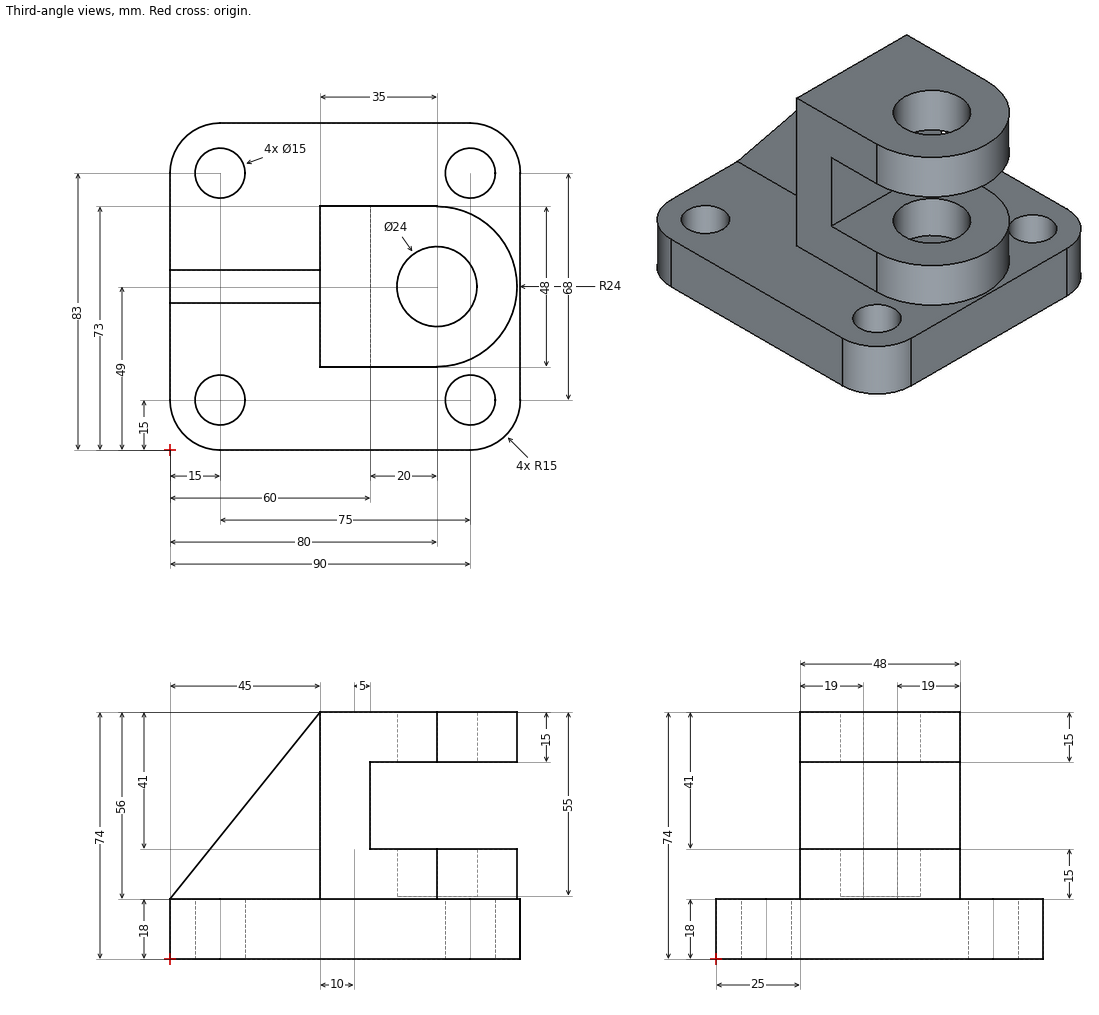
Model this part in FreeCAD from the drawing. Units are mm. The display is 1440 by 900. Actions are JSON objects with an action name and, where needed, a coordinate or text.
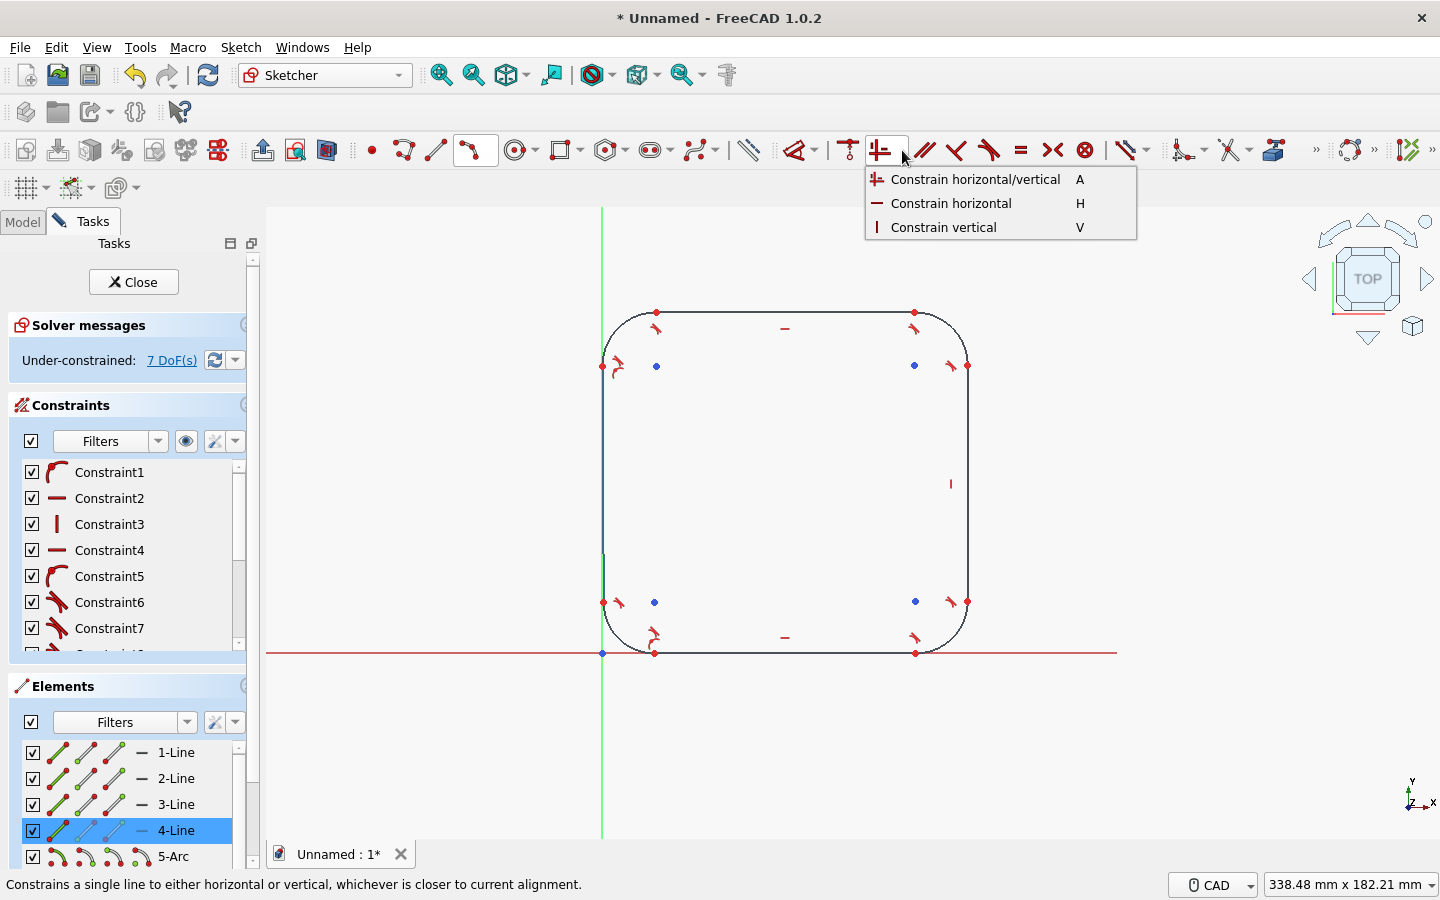
{"action": "left_click", "coordinate": [1001, 227]}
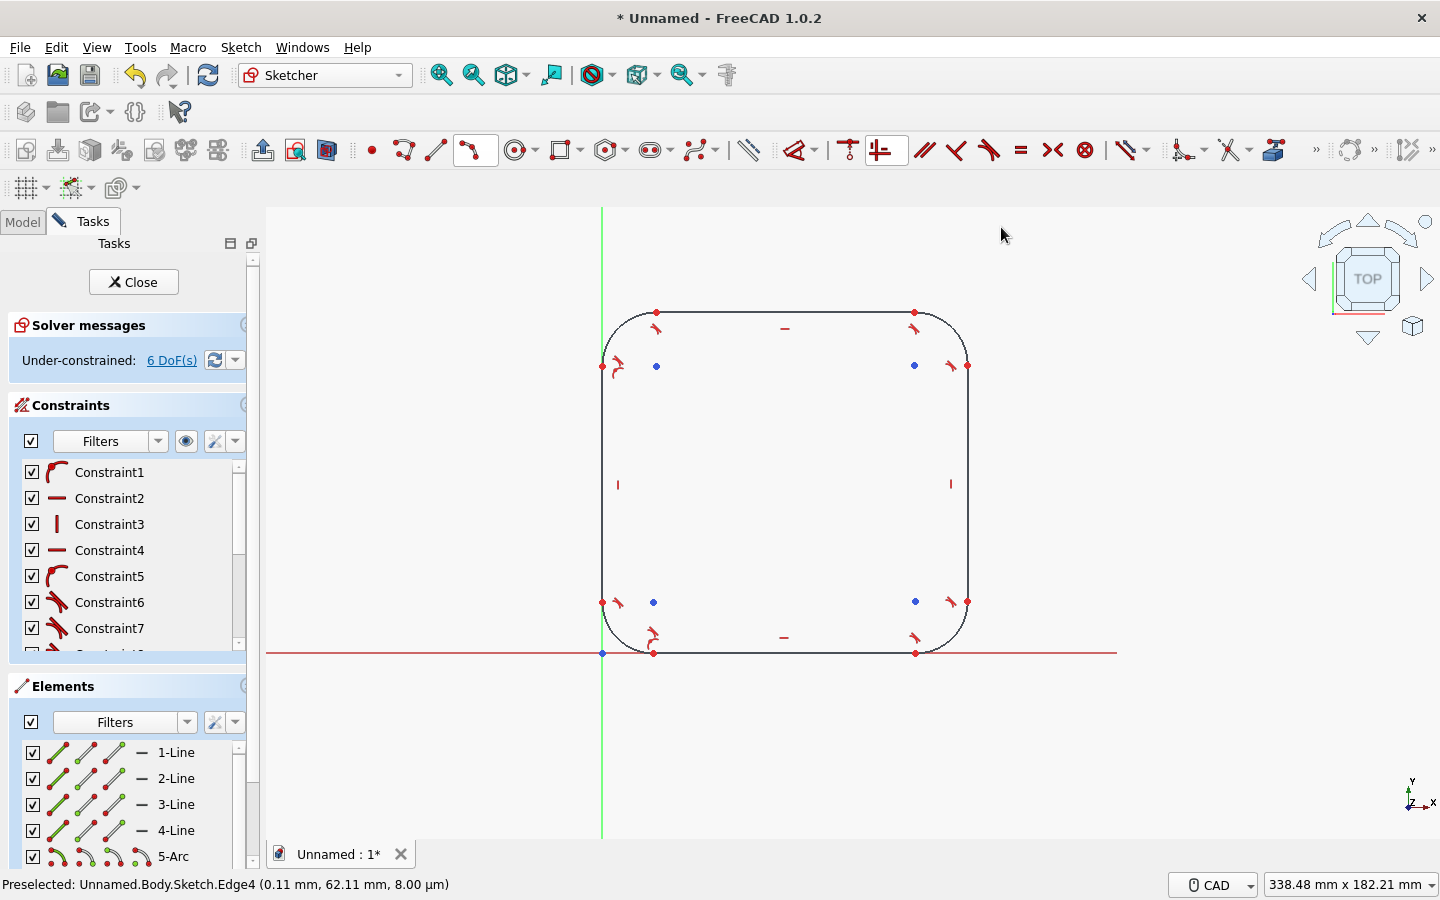
{"action": "left_click", "coordinate": [962, 625]}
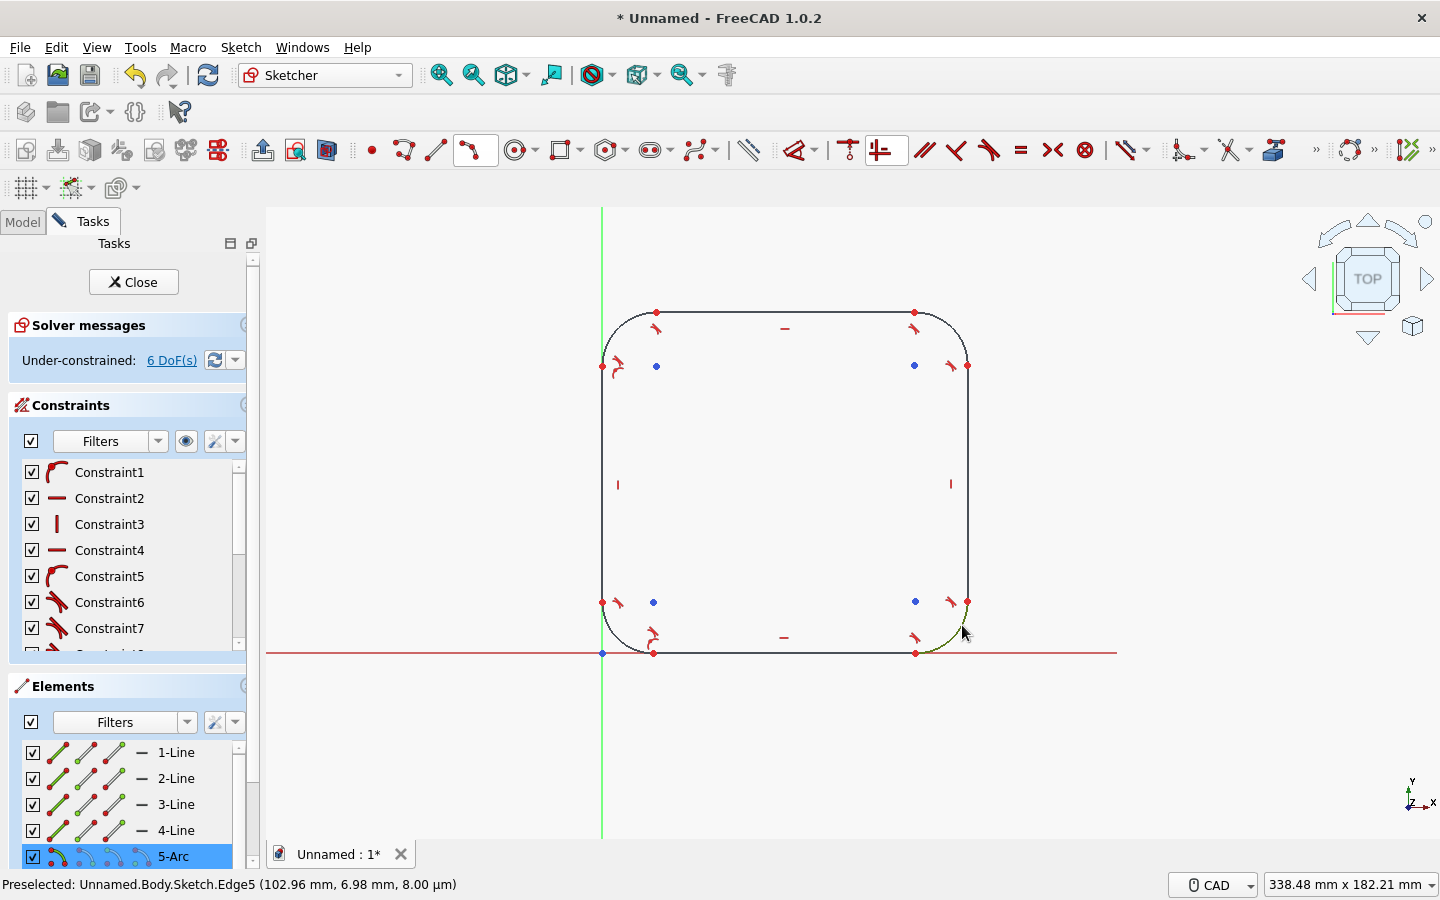
{"action": "left_click", "coordinate": [962, 341]}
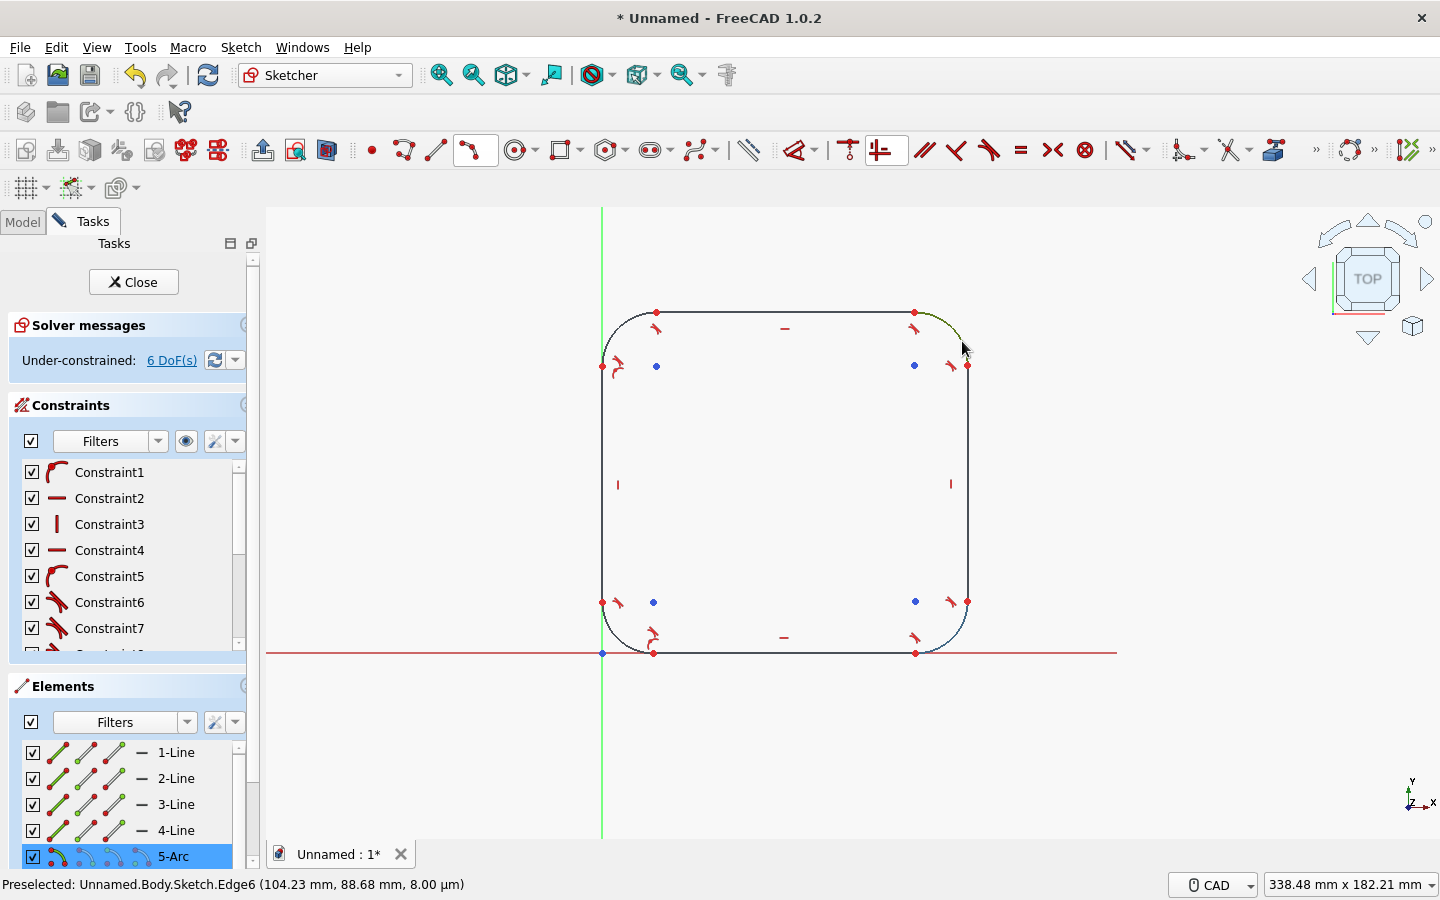
{"action": "left_click", "coordinate": [632, 318]}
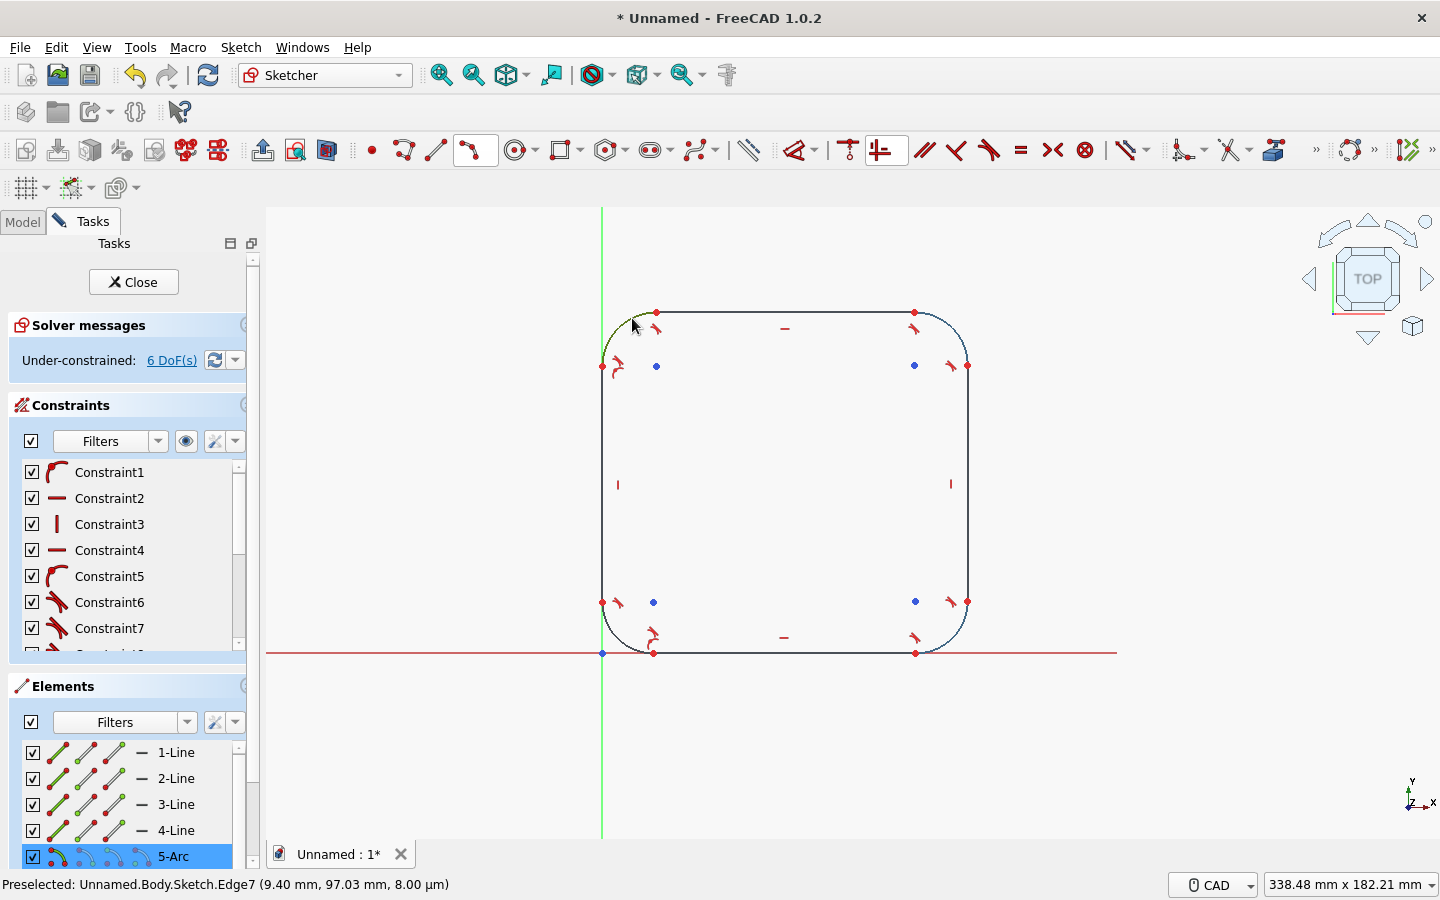
{"action": "left_click", "coordinate": [618, 638]}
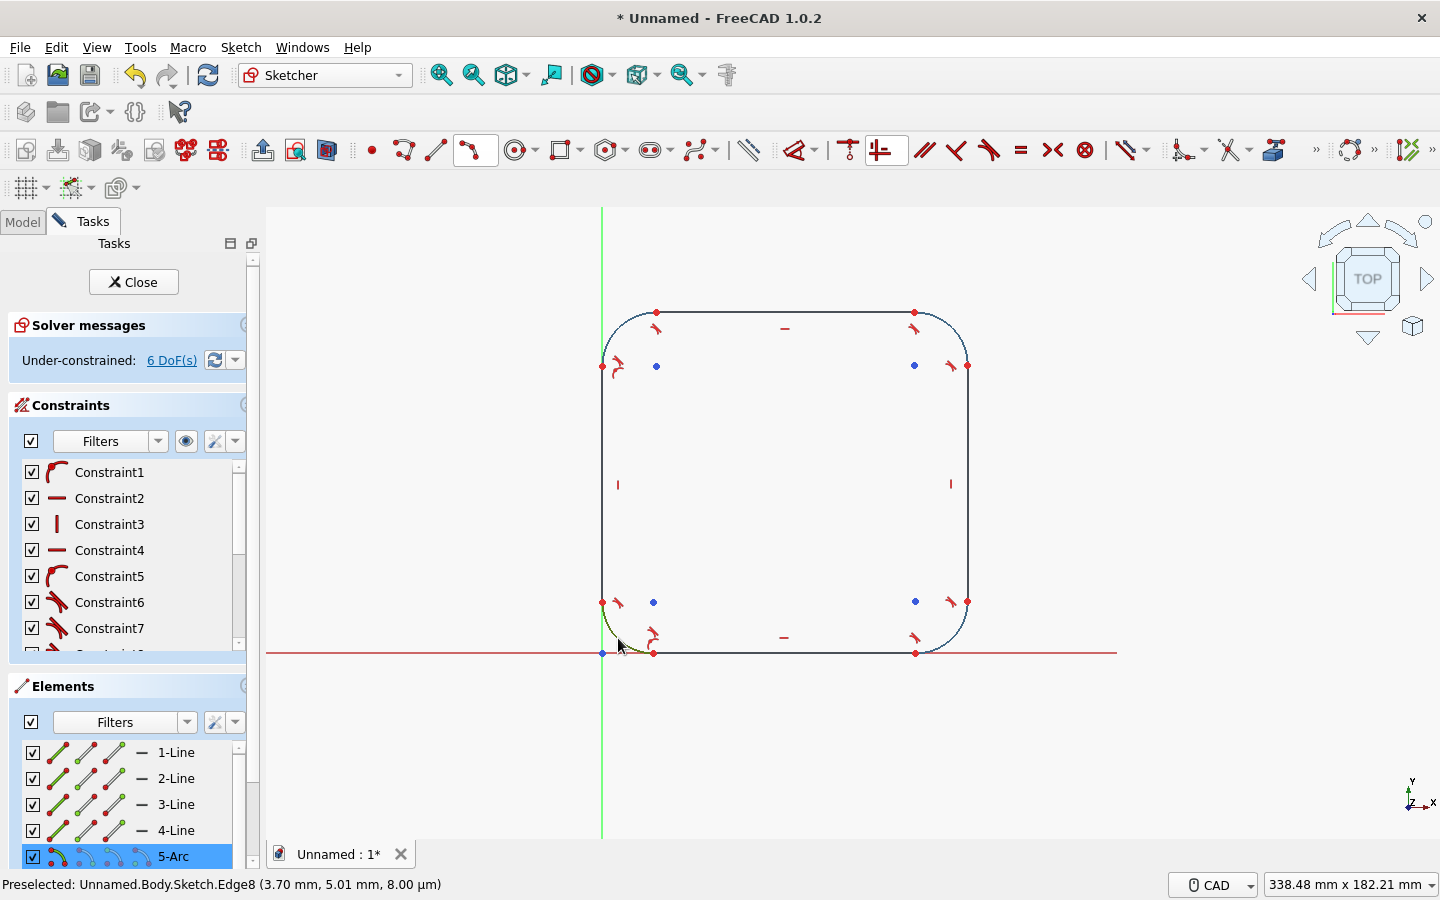
{"action": "left_click", "coordinate": [1022, 150]}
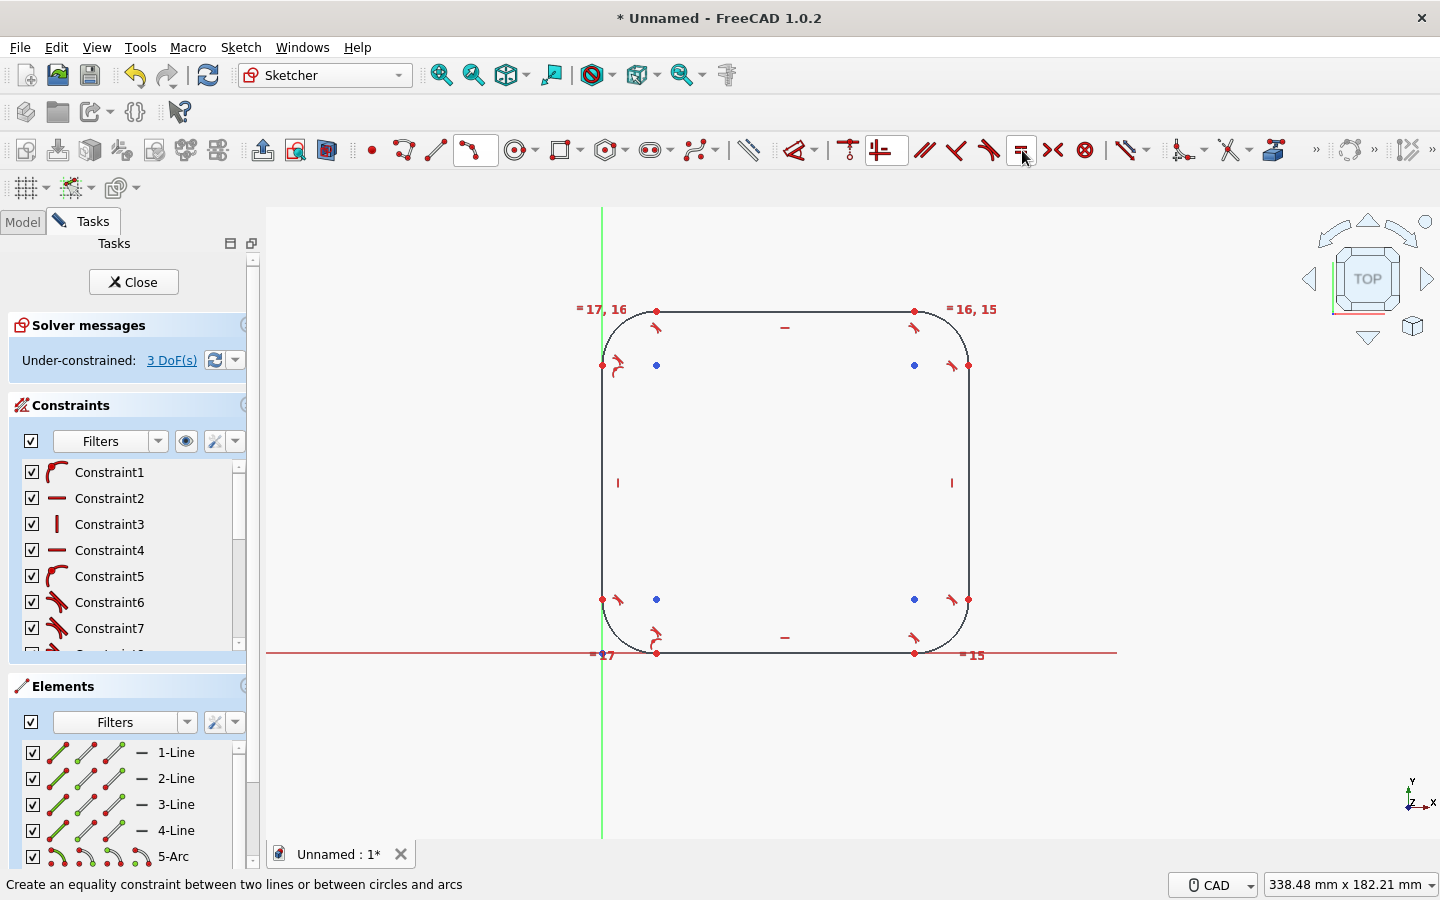
{"action": "left_click", "coordinate": [963, 624]}